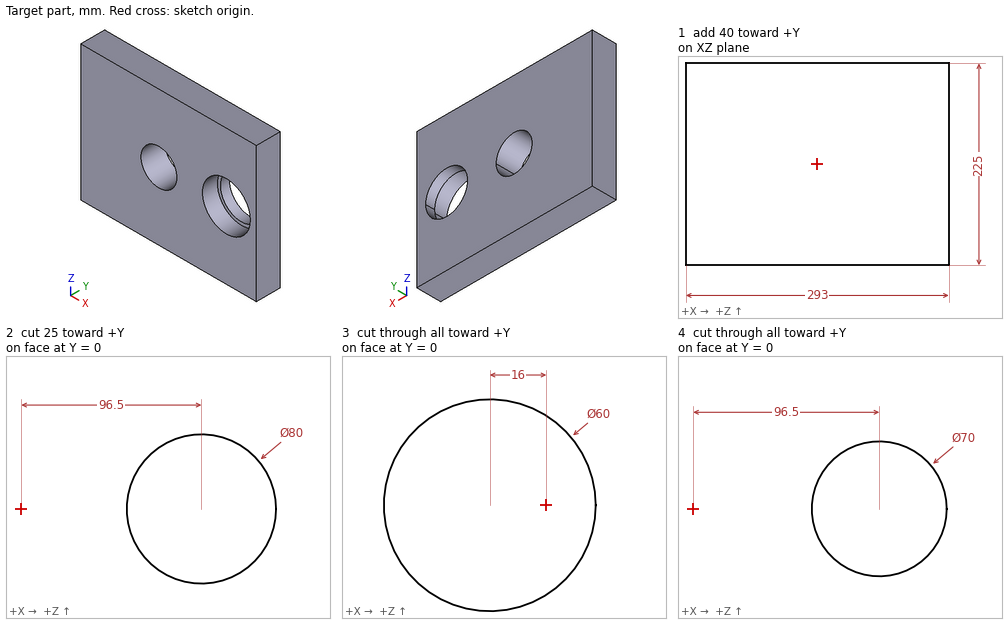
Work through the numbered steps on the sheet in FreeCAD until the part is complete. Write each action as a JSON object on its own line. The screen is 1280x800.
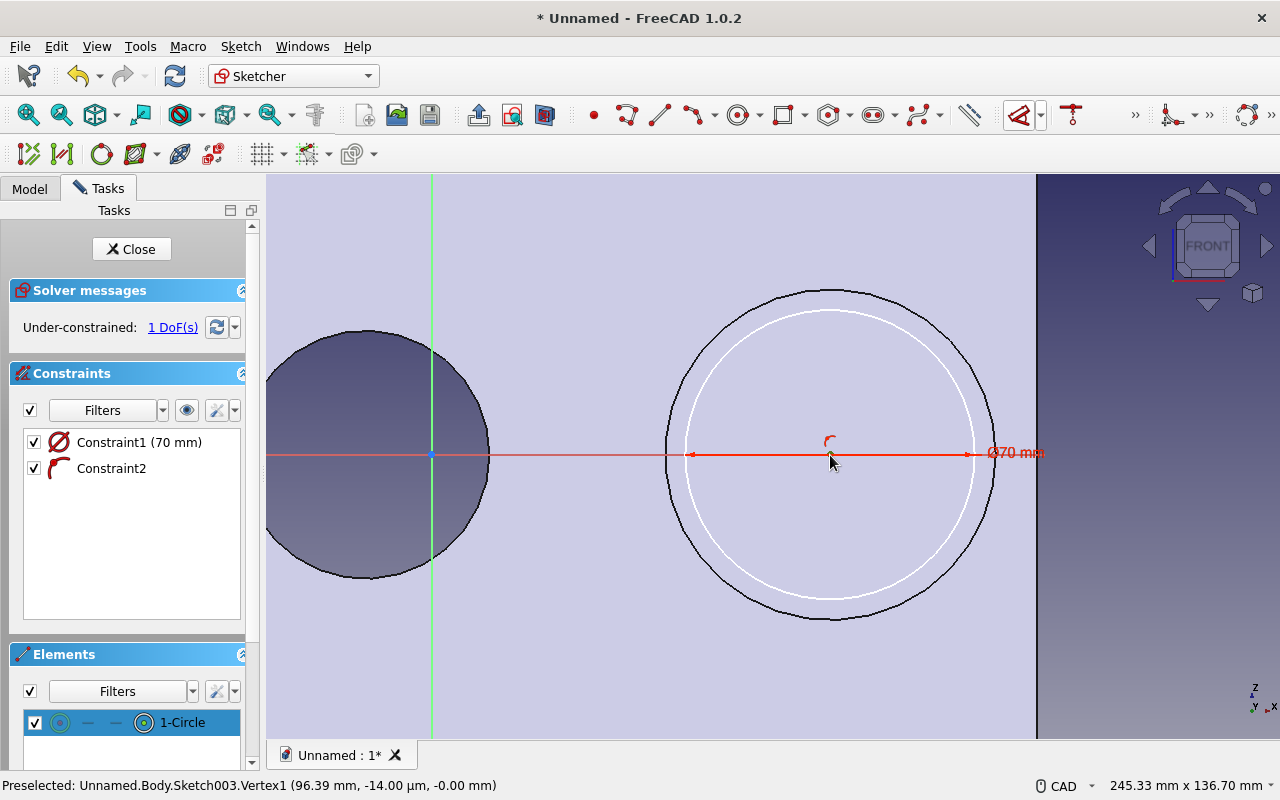
{"action": "left_click", "coordinate": [1040, 116]}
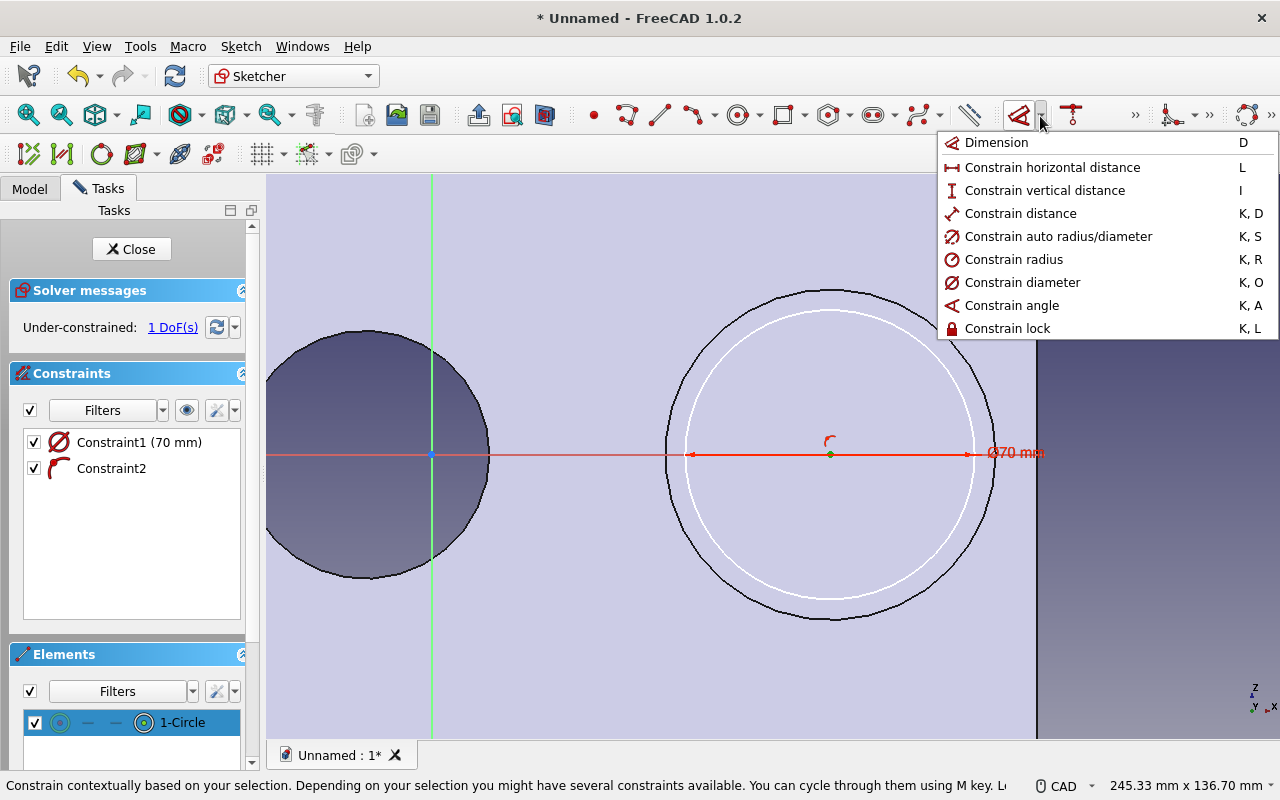
{"action": "left_click", "coordinate": [1108, 168]}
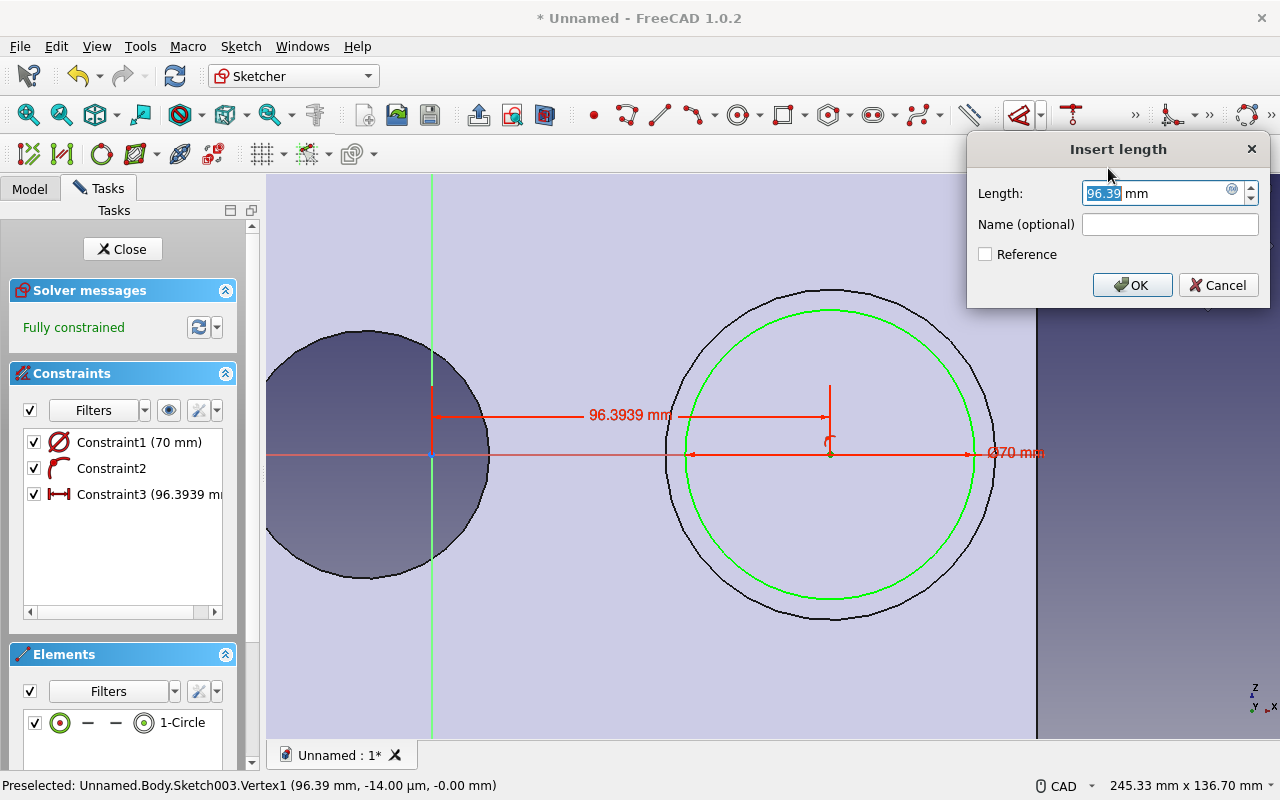
{"action": "type", "text": "96.5"}
{"action": "key", "text": "Return"}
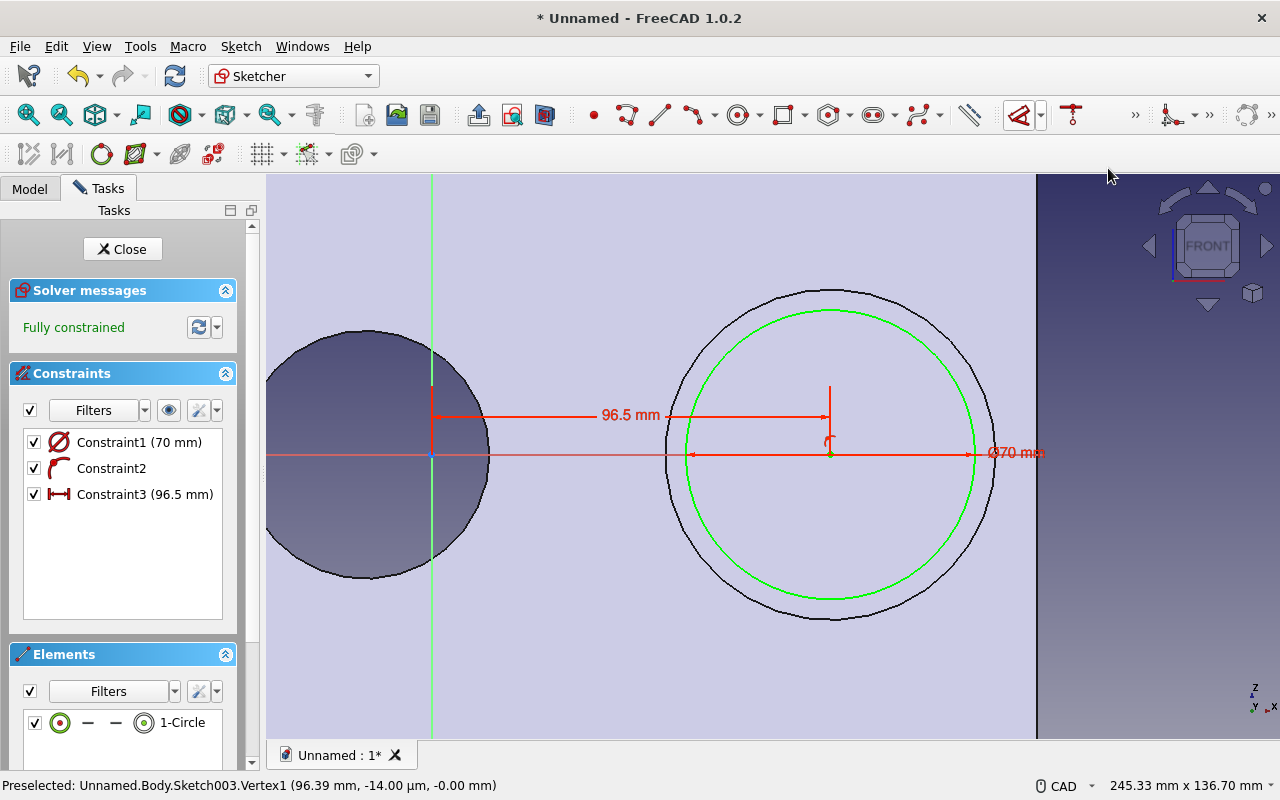
{"action": "left_click", "coordinate": [123, 249]}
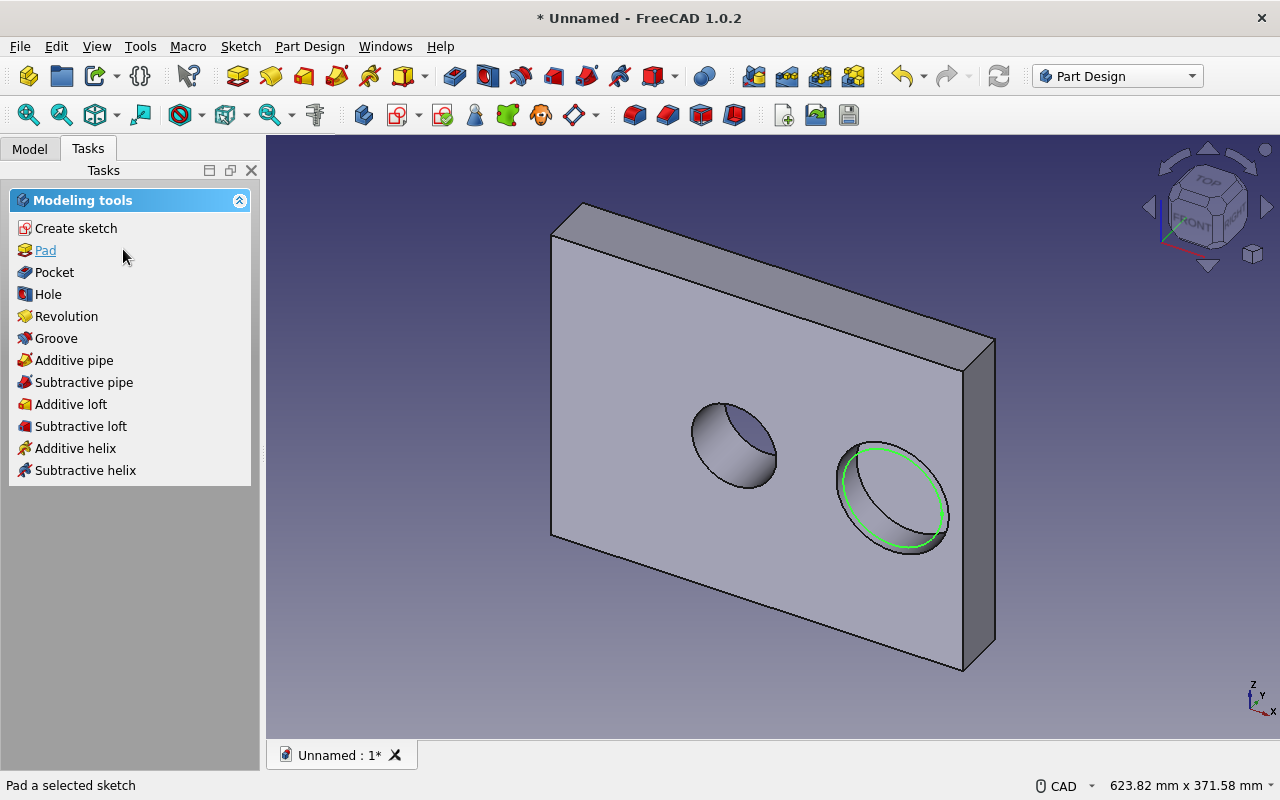
{"action": "left_click", "coordinate": [455, 76]}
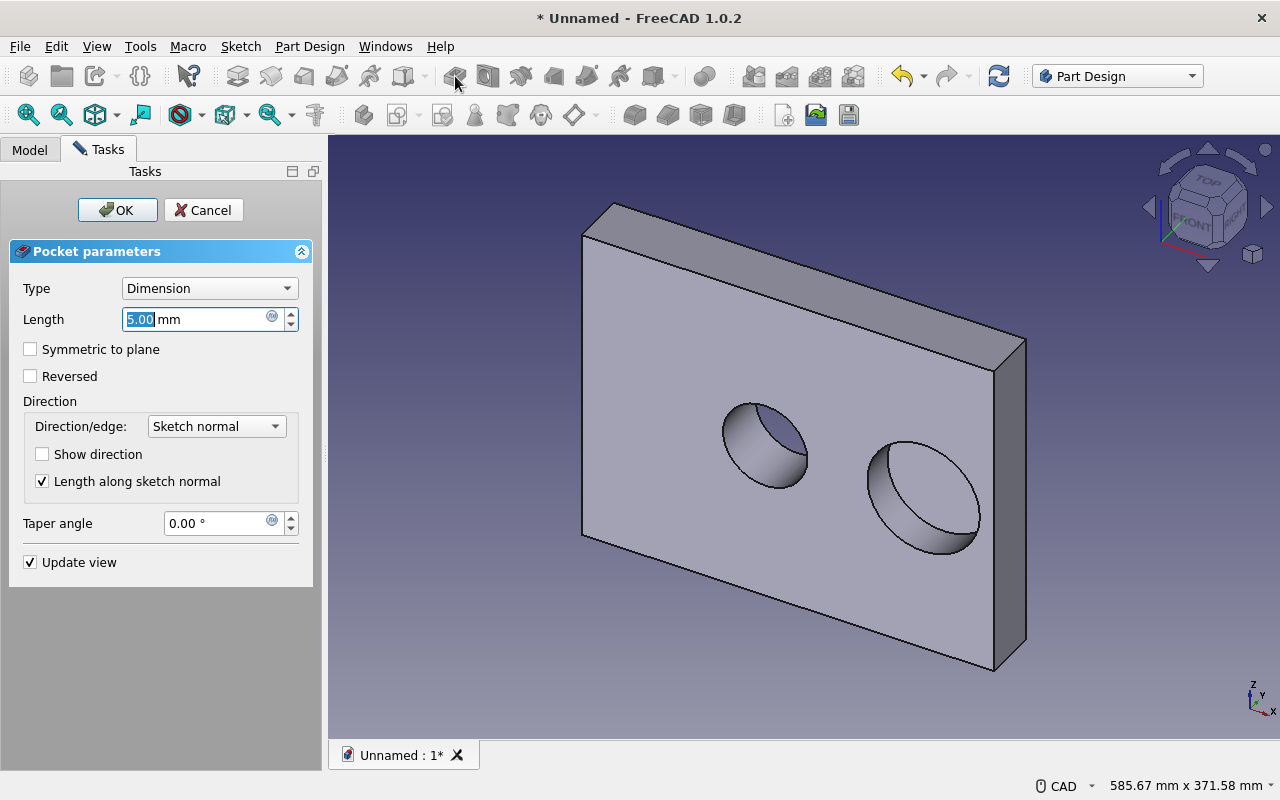
{"action": "left_click", "coordinate": [210, 288]}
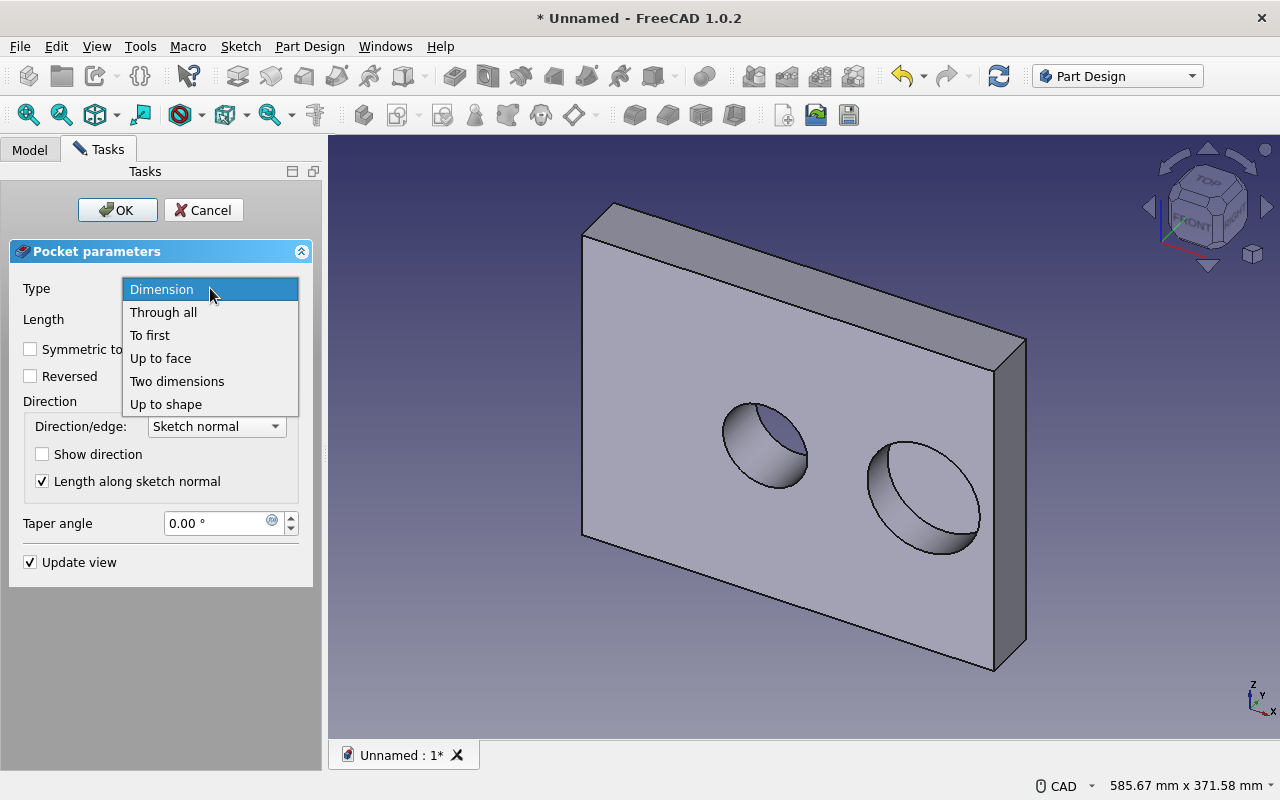
{"action": "left_click", "coordinate": [208, 312]}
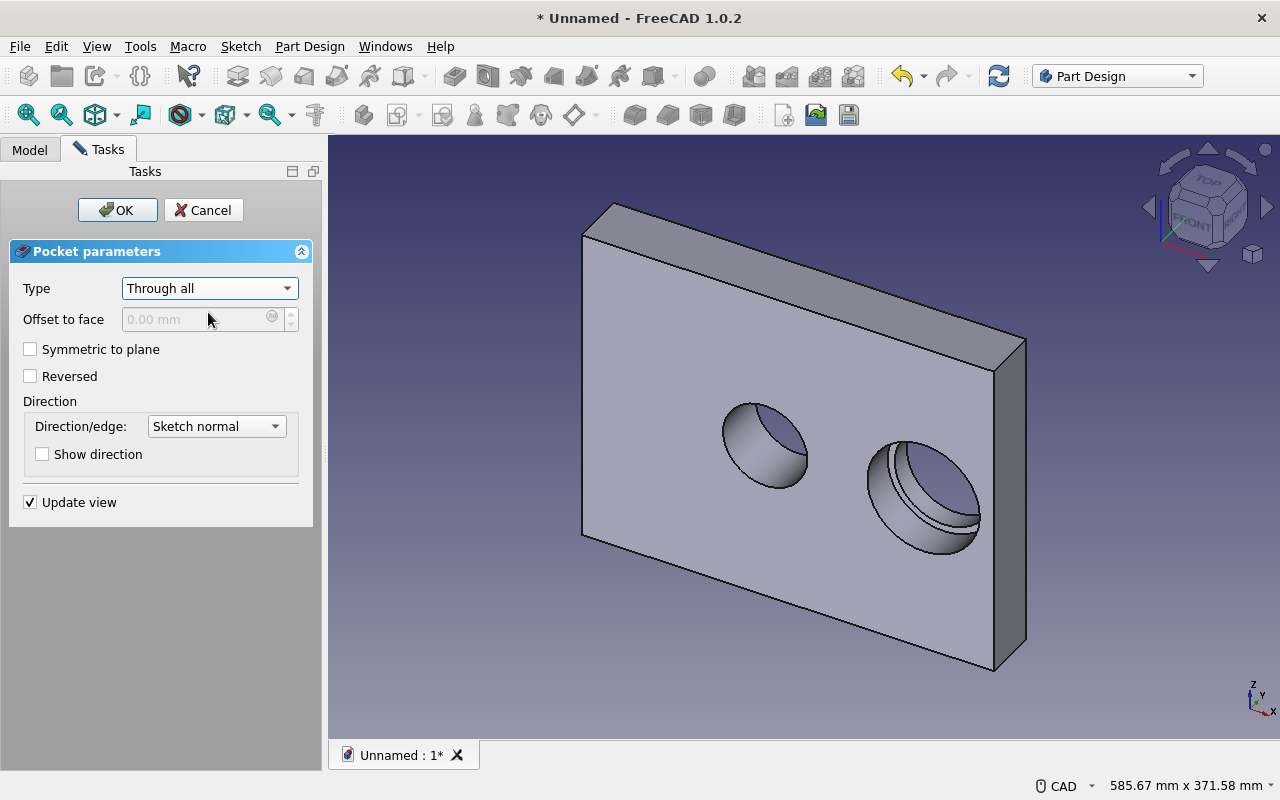
{"action": "left_click", "coordinate": [118, 210]}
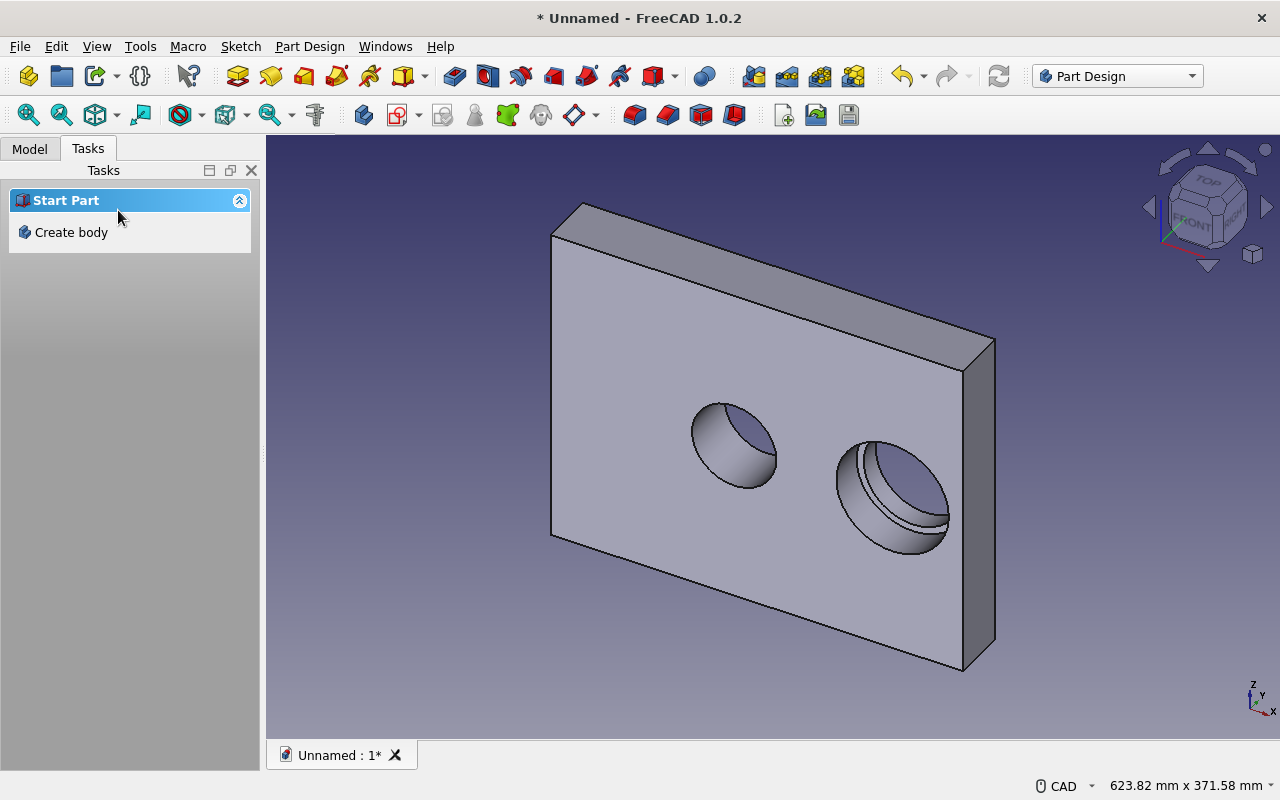
{"action": "key", "text": "0"}